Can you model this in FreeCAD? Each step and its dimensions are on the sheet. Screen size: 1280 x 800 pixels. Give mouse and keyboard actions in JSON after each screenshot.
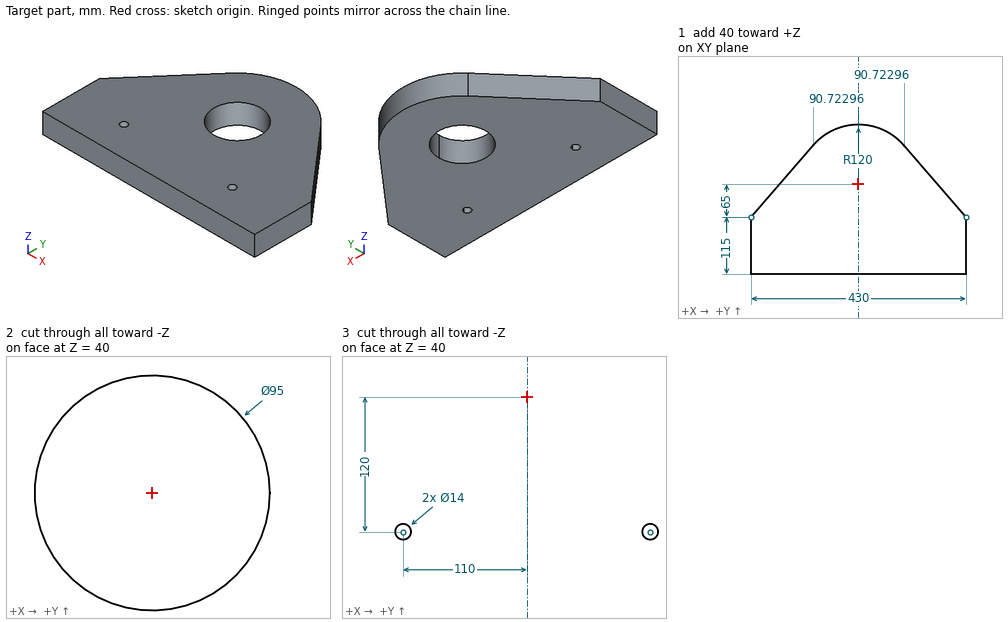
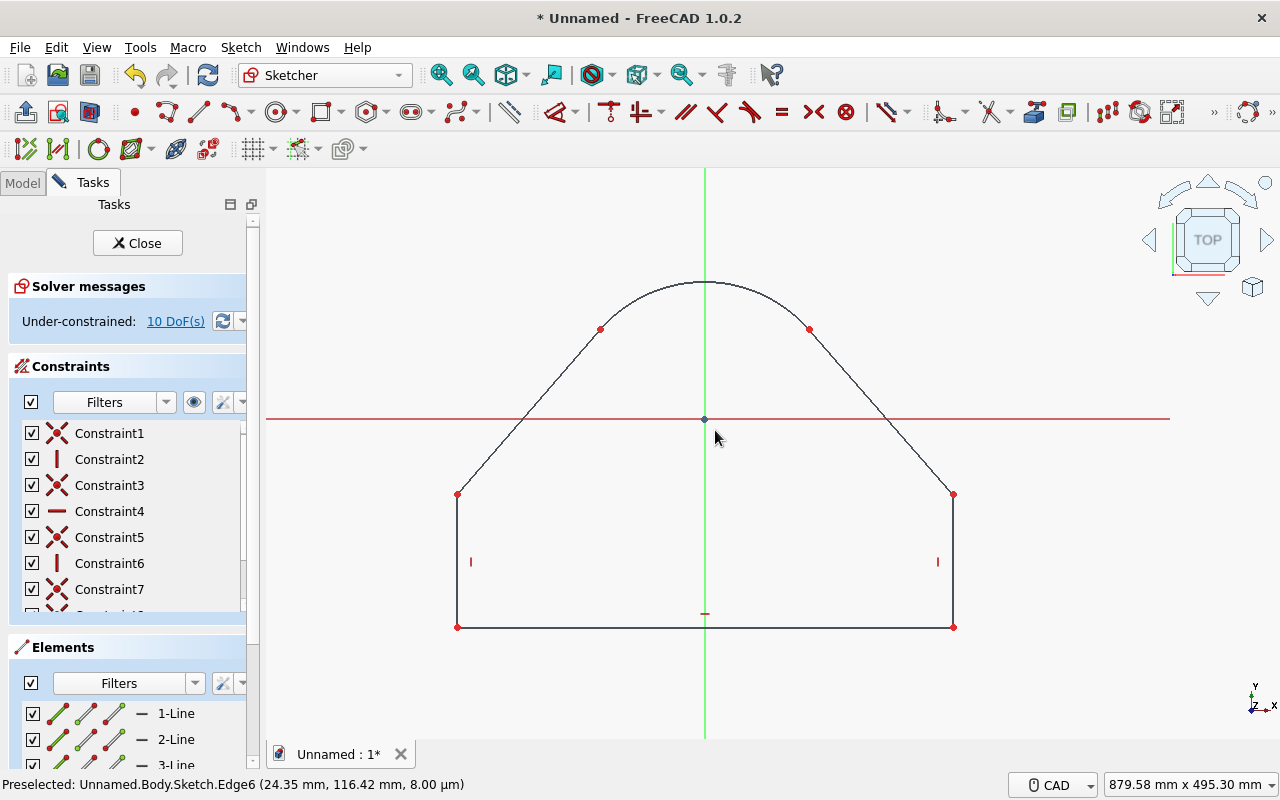
{"action": "left_click", "coordinate": [610, 112]}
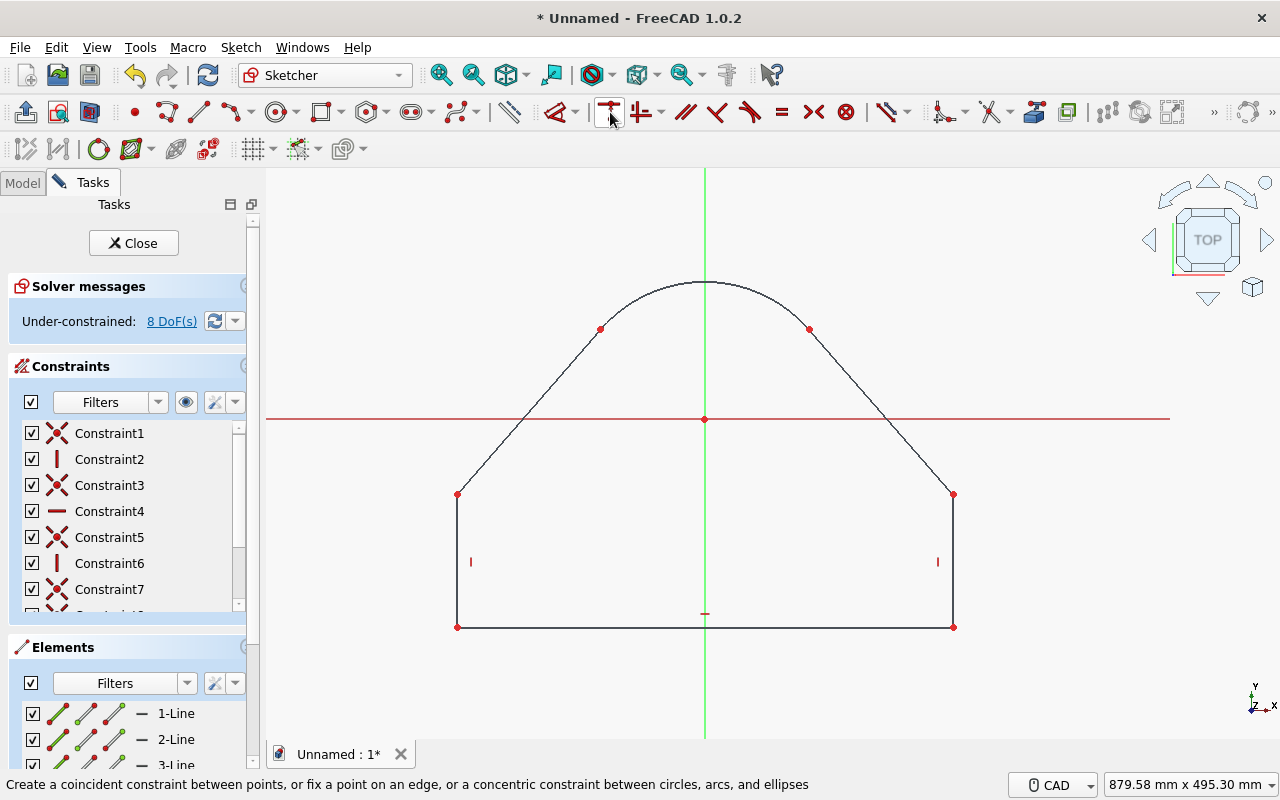
{"action": "left_click", "coordinate": [457, 495]}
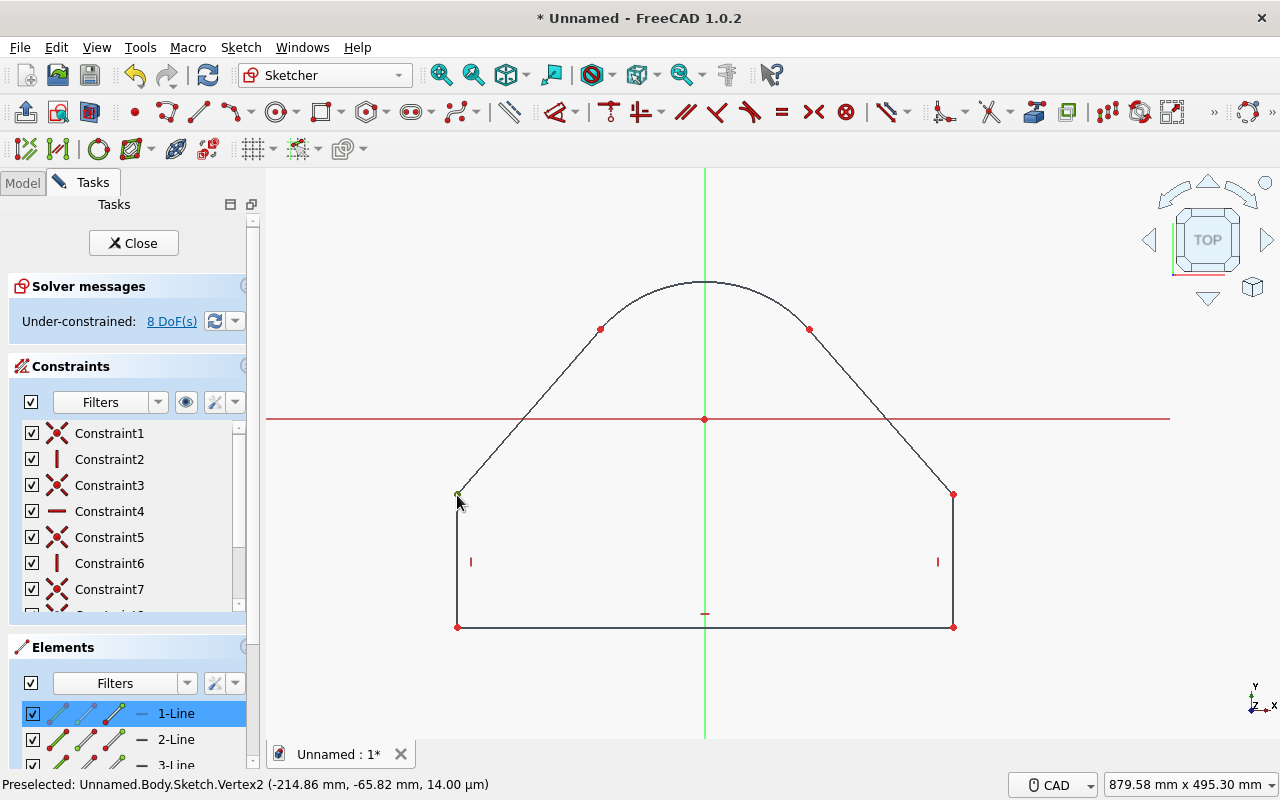
{"action": "left_click", "coordinate": [953, 495]}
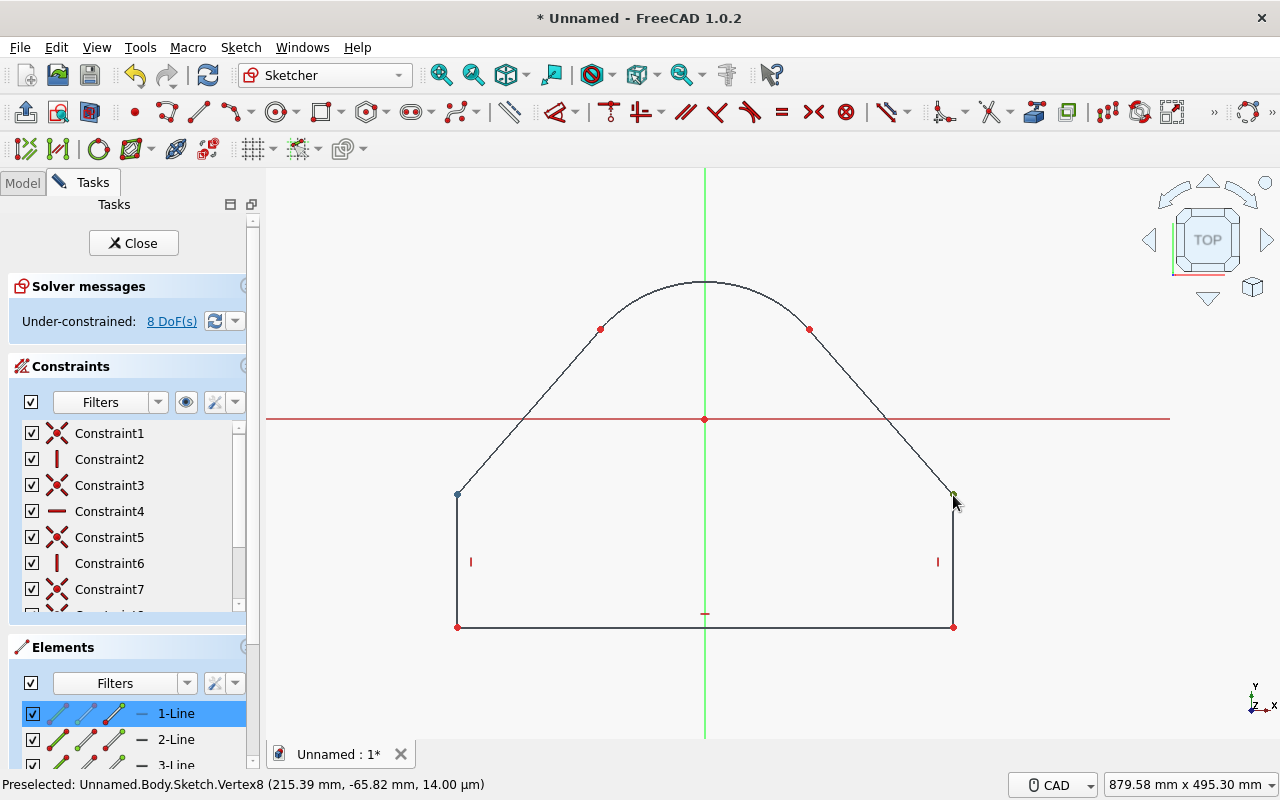
{"action": "left_click", "coordinate": [705, 674]}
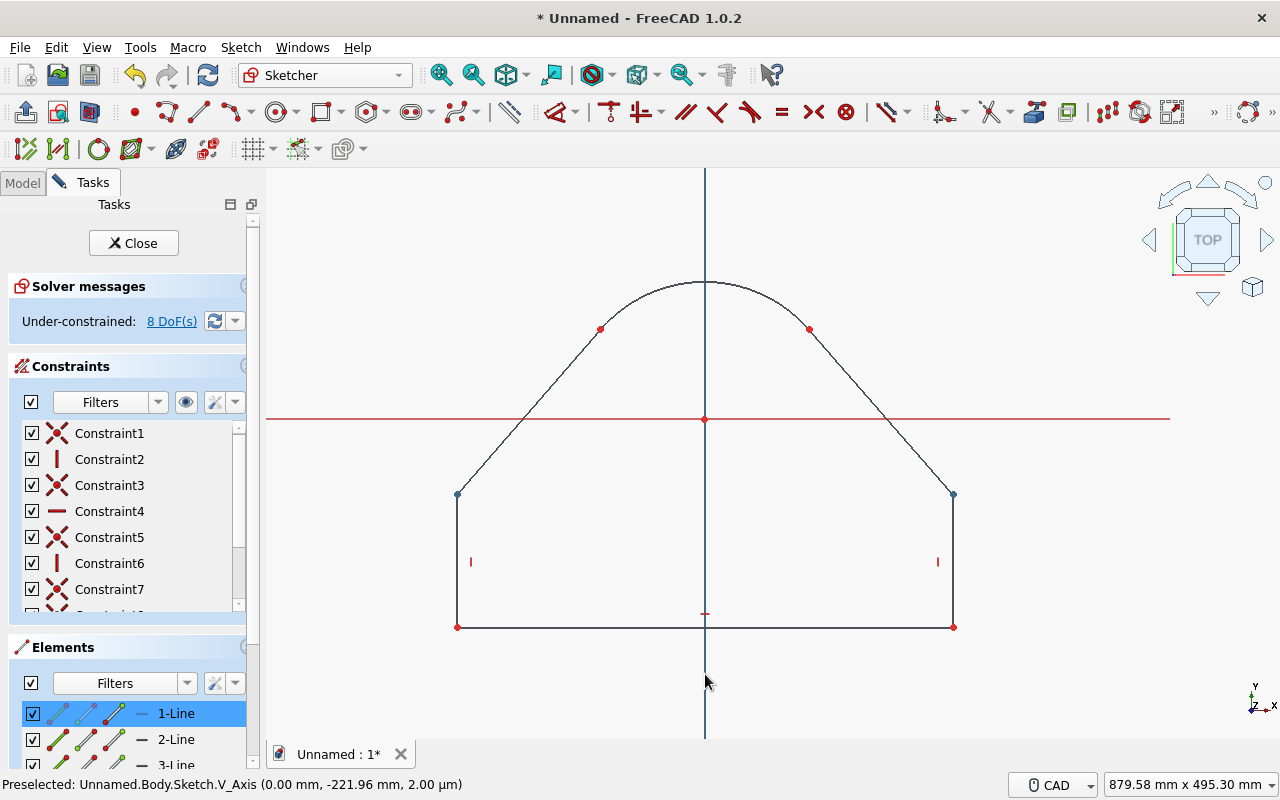
{"action": "left_click", "coordinate": [814, 112]}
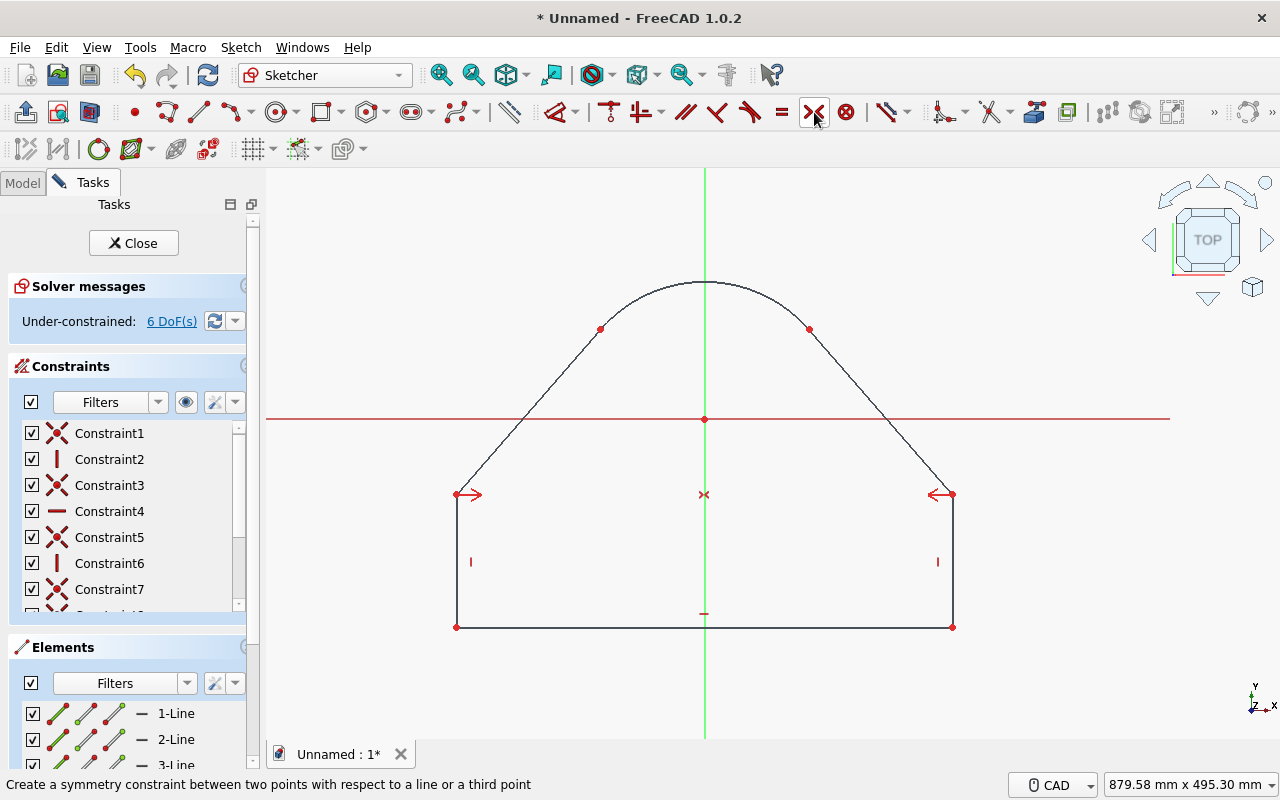
{"action": "left_click", "coordinate": [556, 112]}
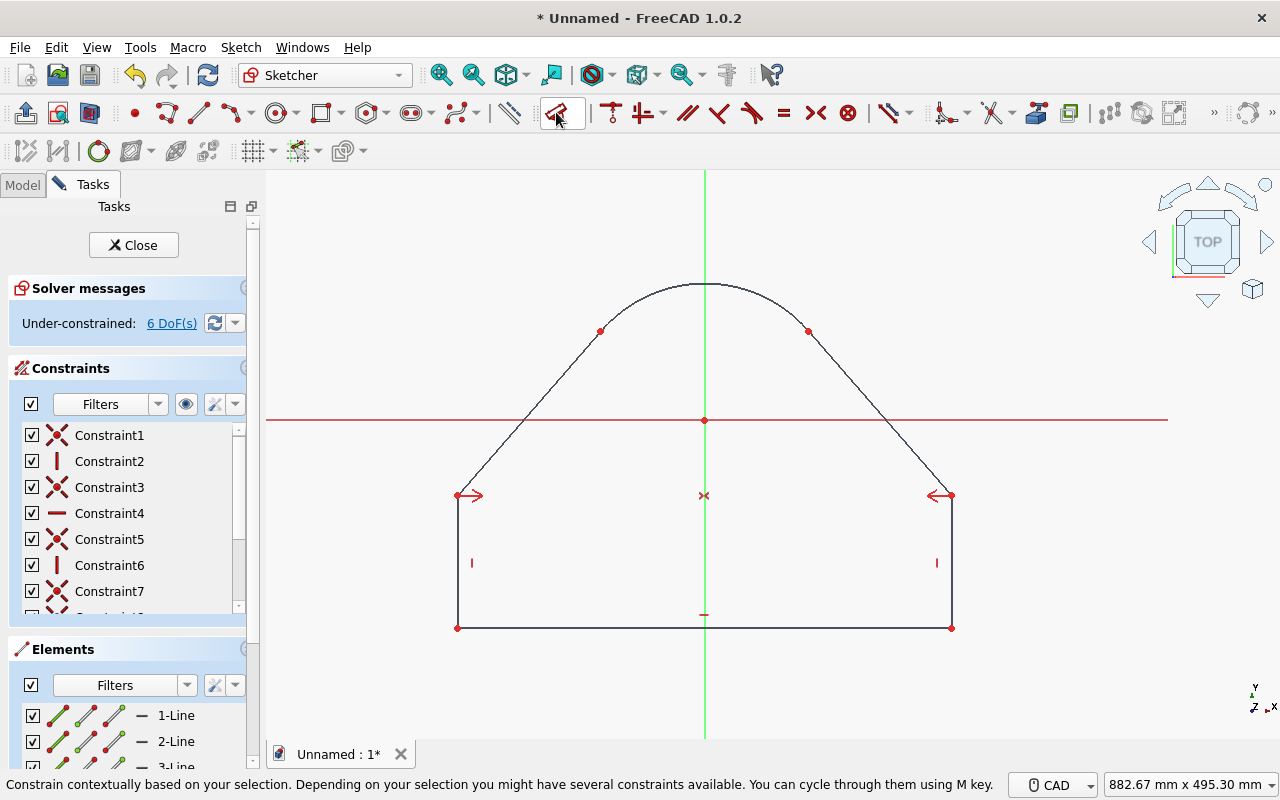
{"action": "left_click", "coordinate": [751, 292]}
{"action": "left_click", "coordinate": [762, 262]}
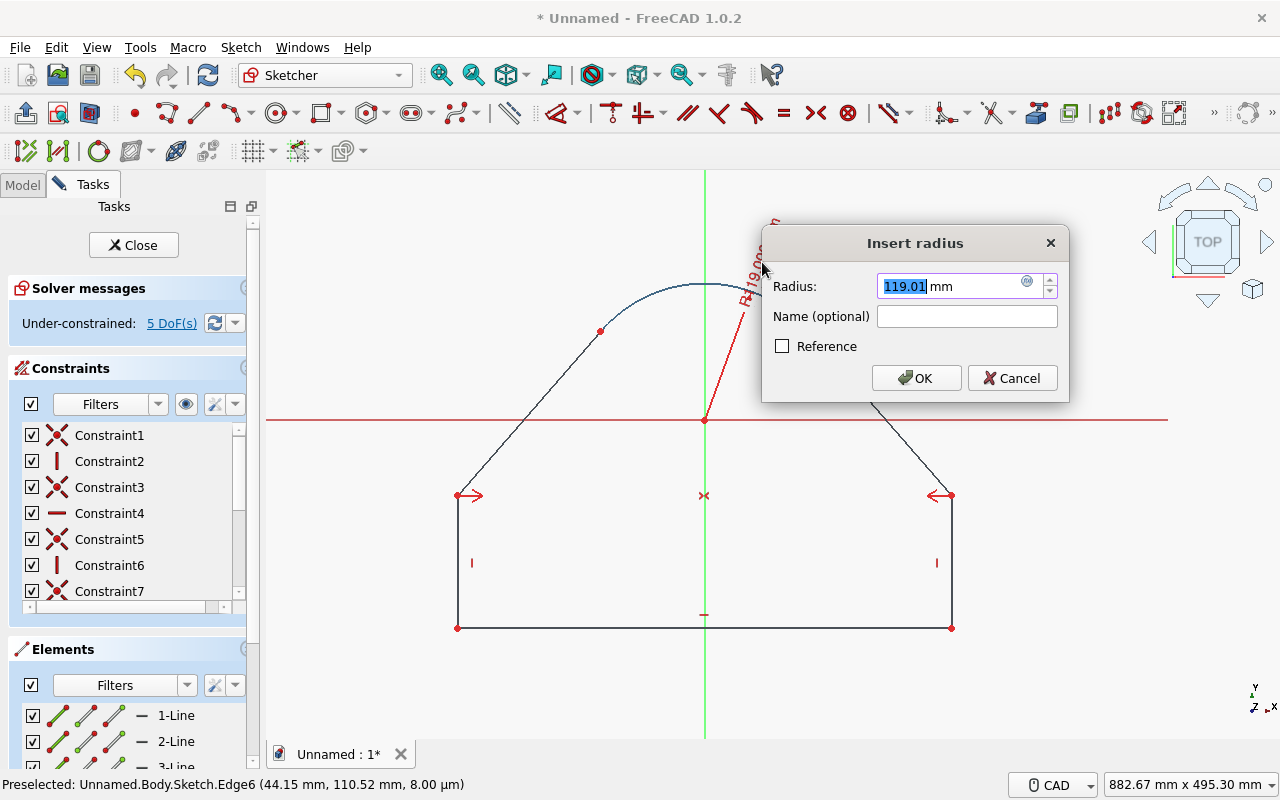
{"action": "type", "text": "120"}
{"action": "key", "text": "Return"}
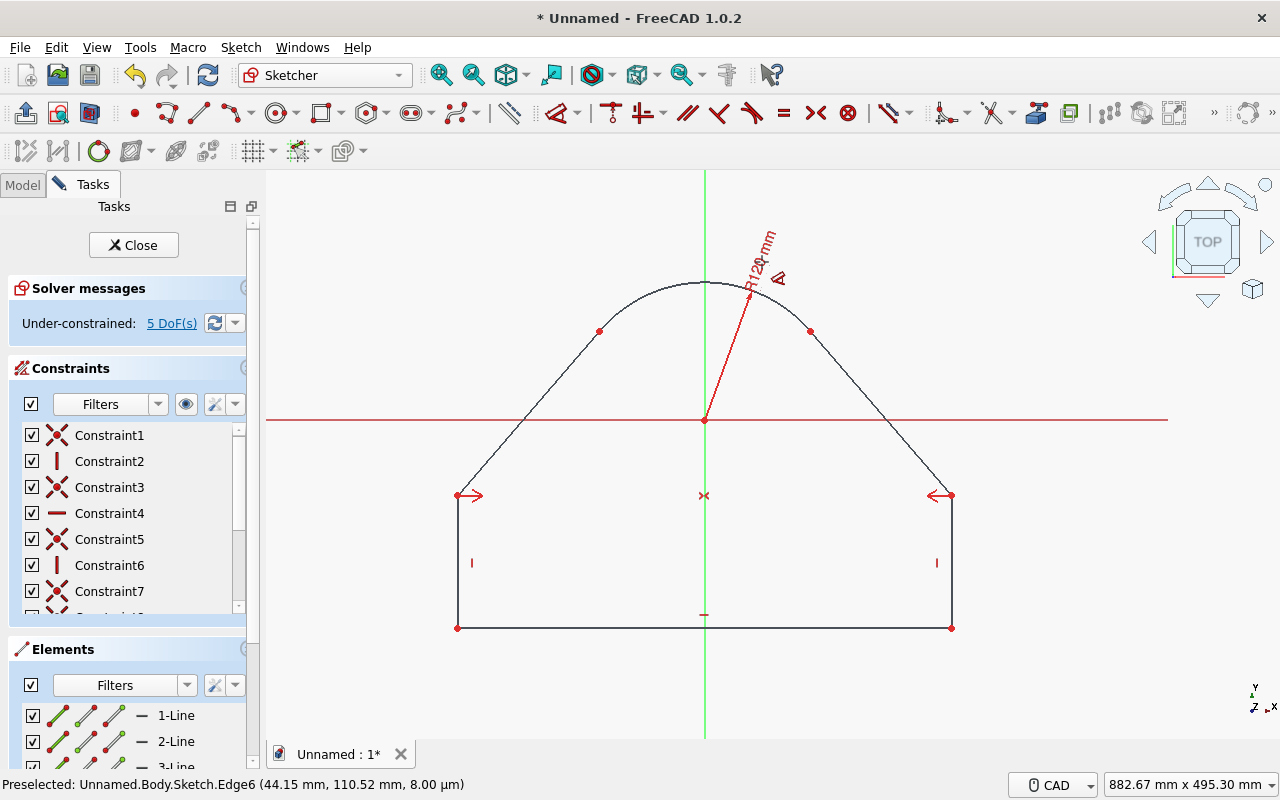
{"action": "left_click", "coordinate": [458, 536]}
{"action": "left_click", "coordinate": [424, 562]}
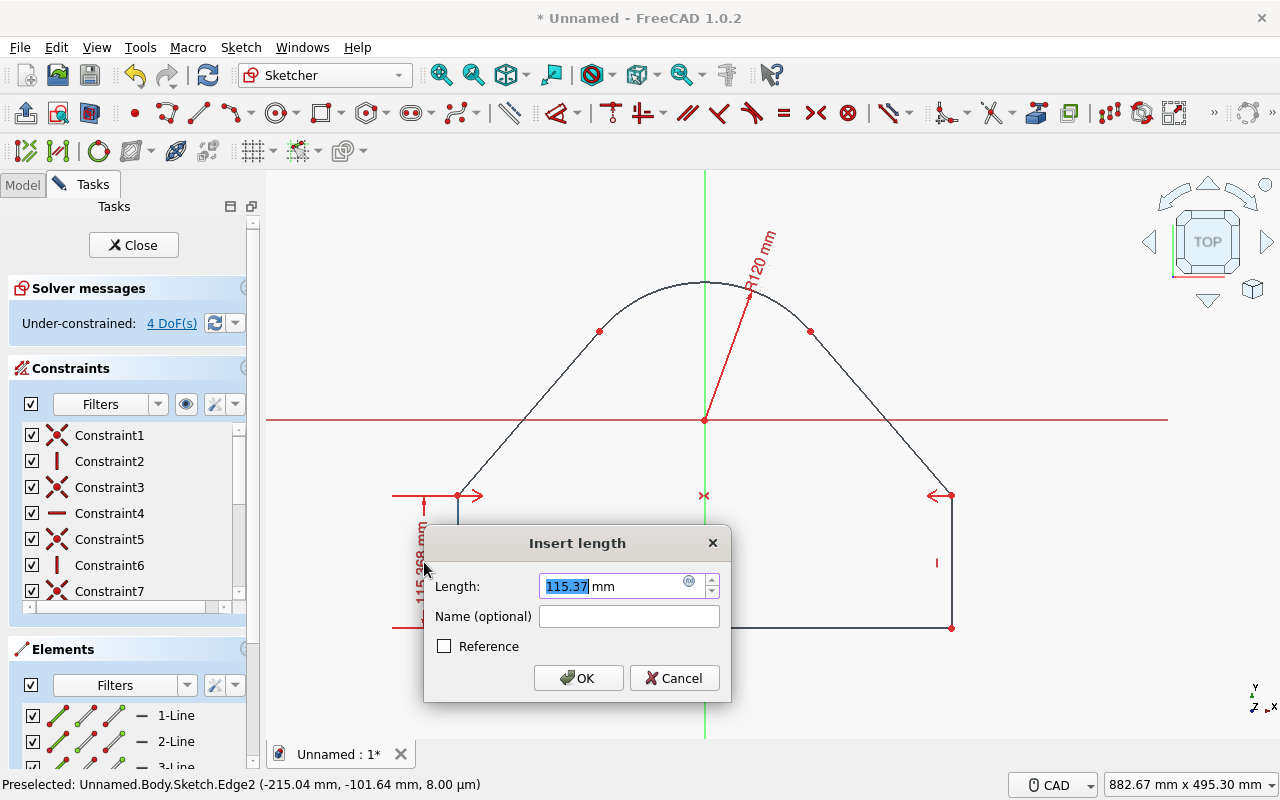
{"action": "type", "text": "115"}
{"action": "key", "text": "Return"}